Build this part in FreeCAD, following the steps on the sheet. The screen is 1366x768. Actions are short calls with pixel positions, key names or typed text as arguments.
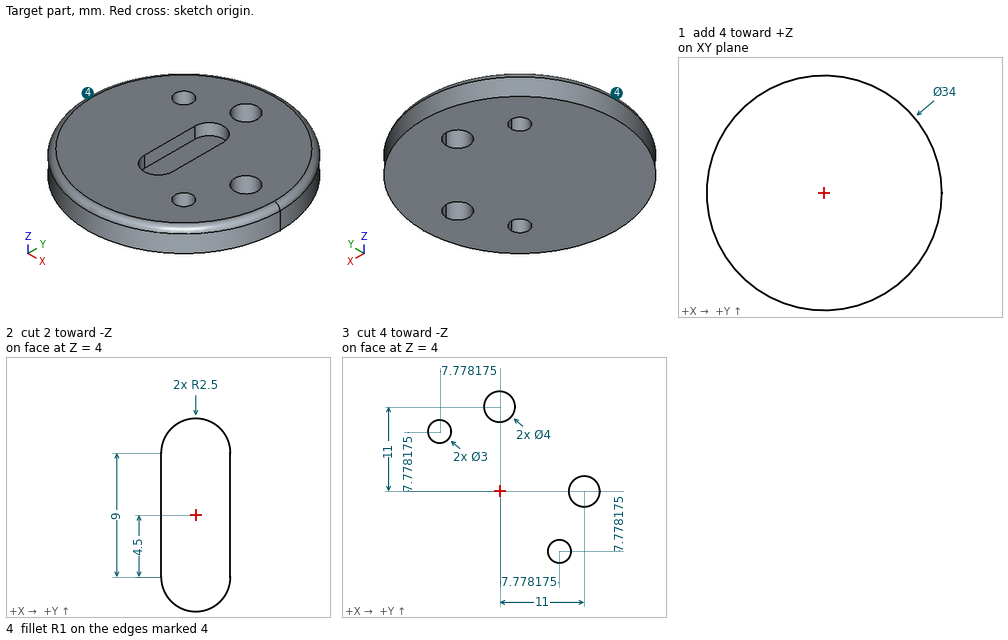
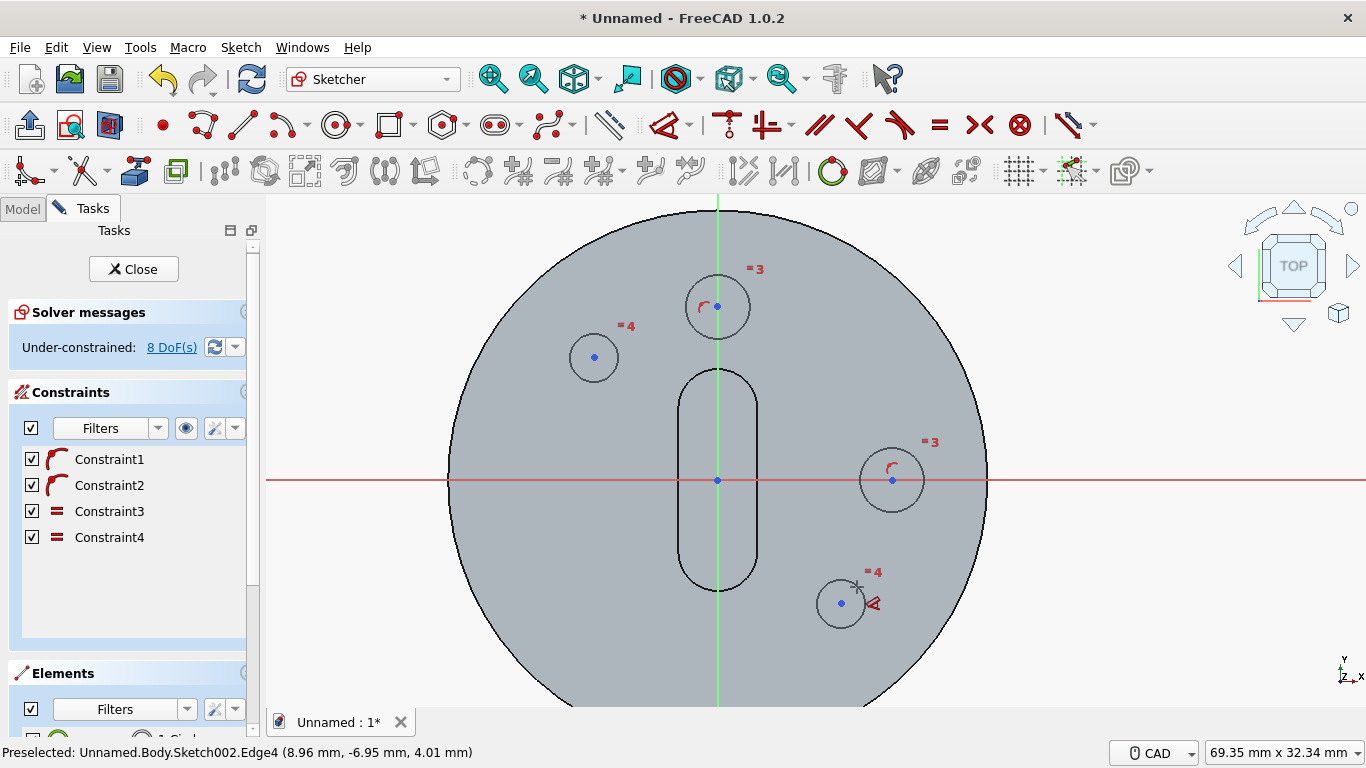
click(740, 284)
click(762, 261)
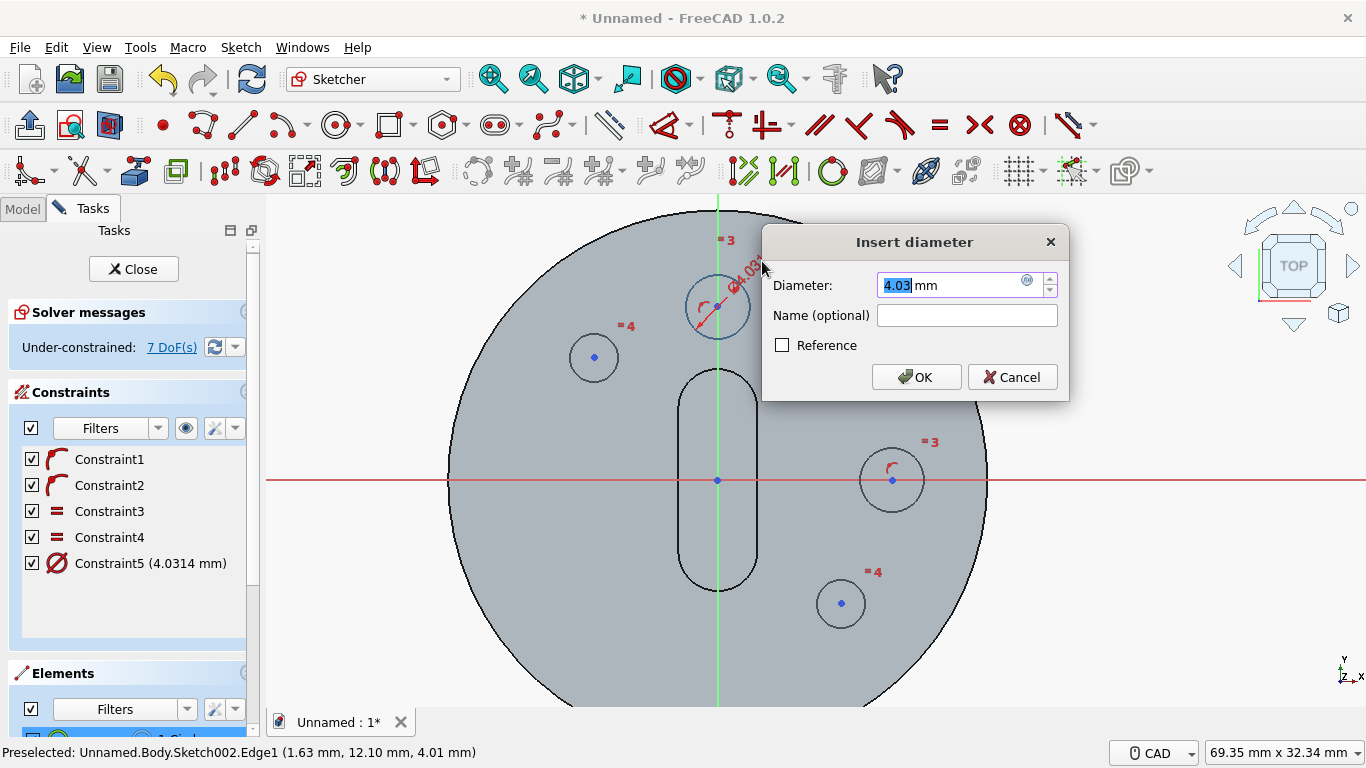
text(4)
key(Return)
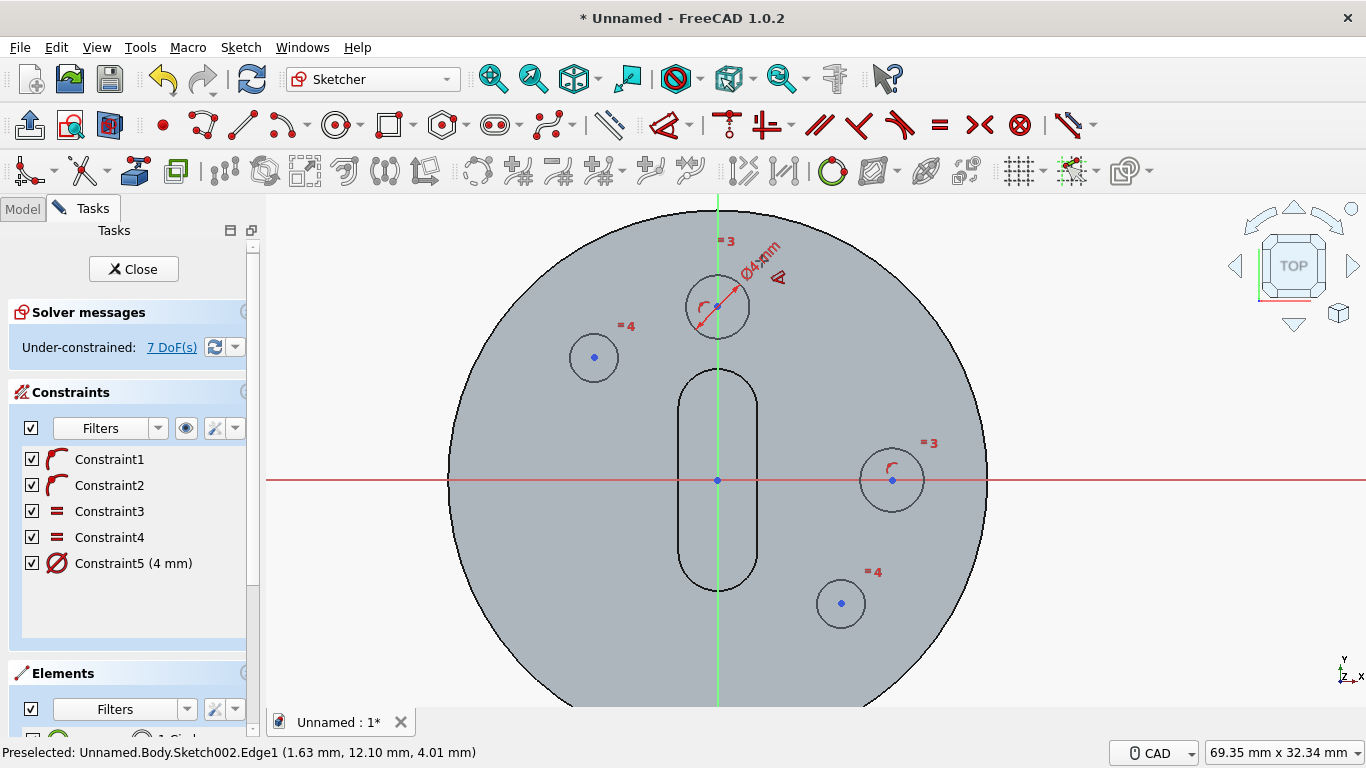
click(611, 341)
click(634, 318)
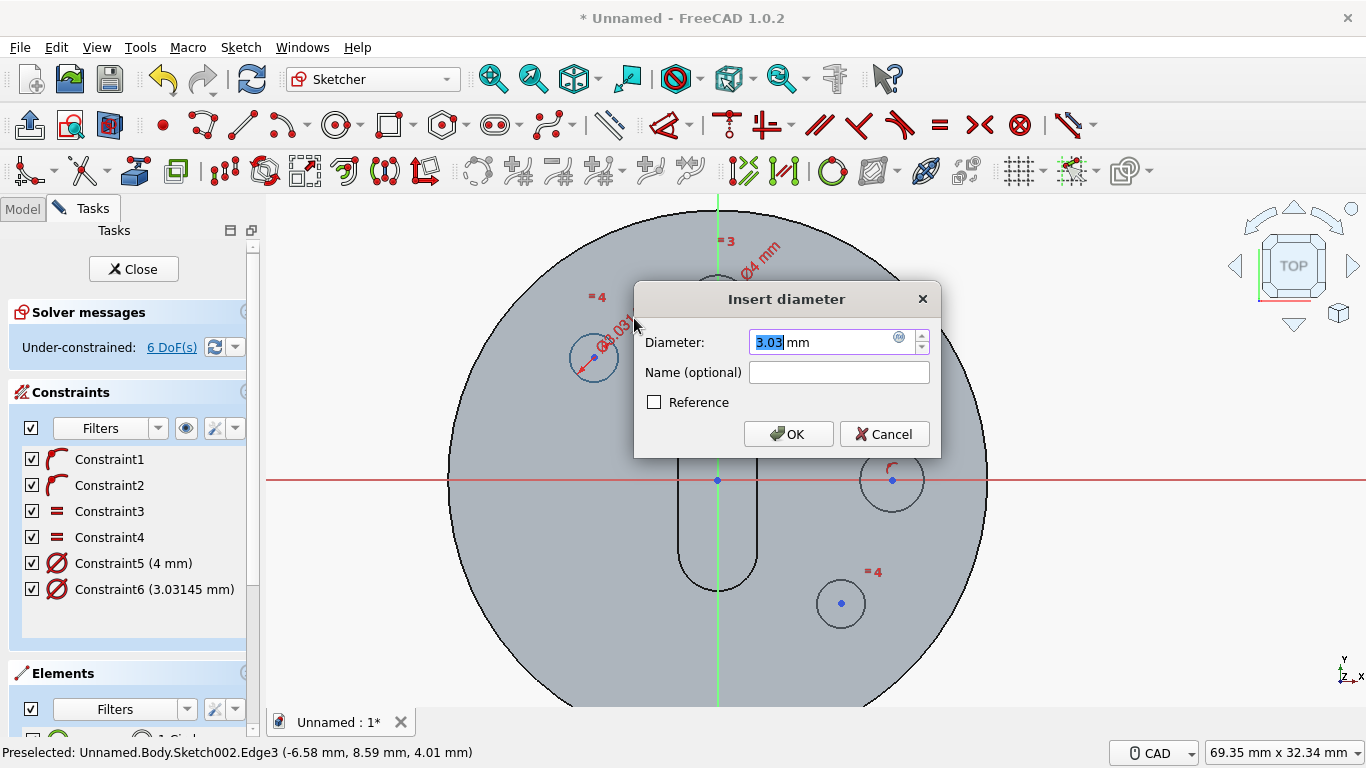
text(3)
key(Return)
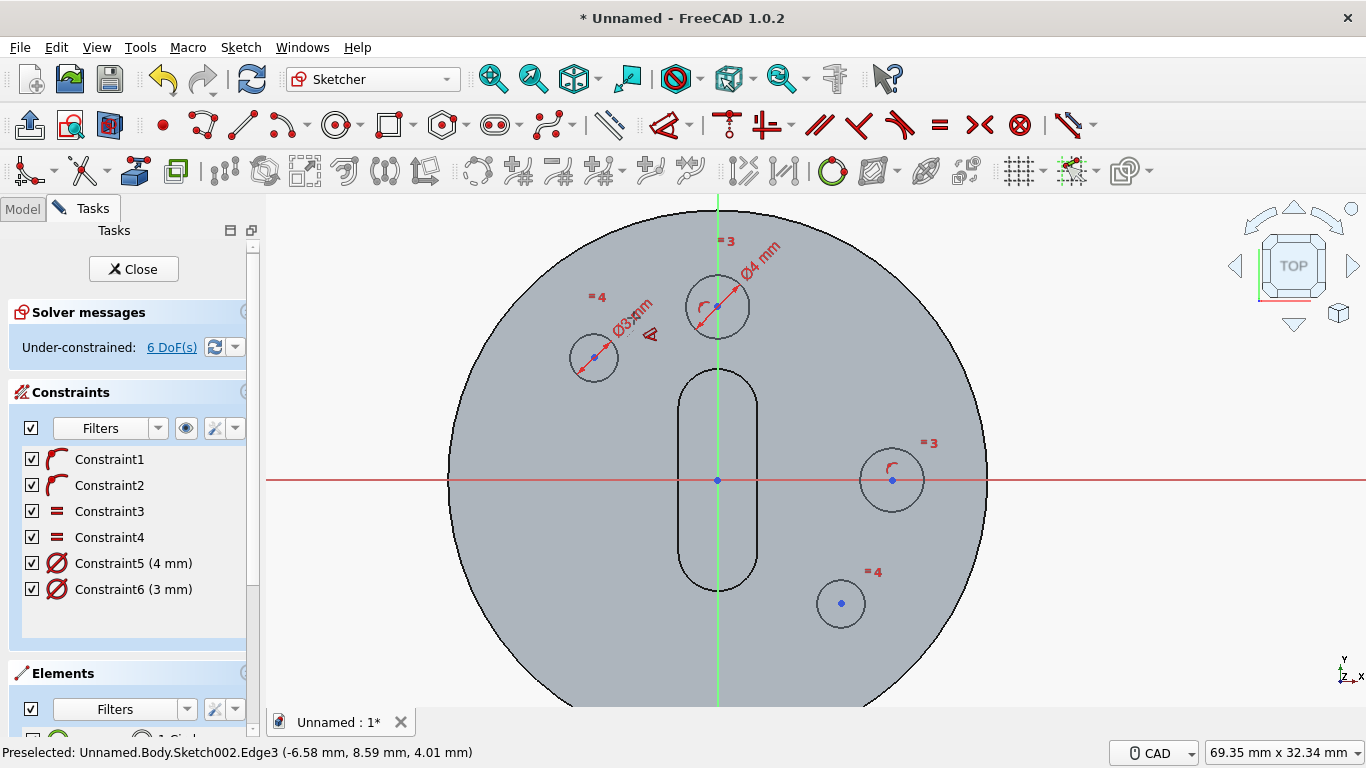
click(718, 307)
click(684, 394)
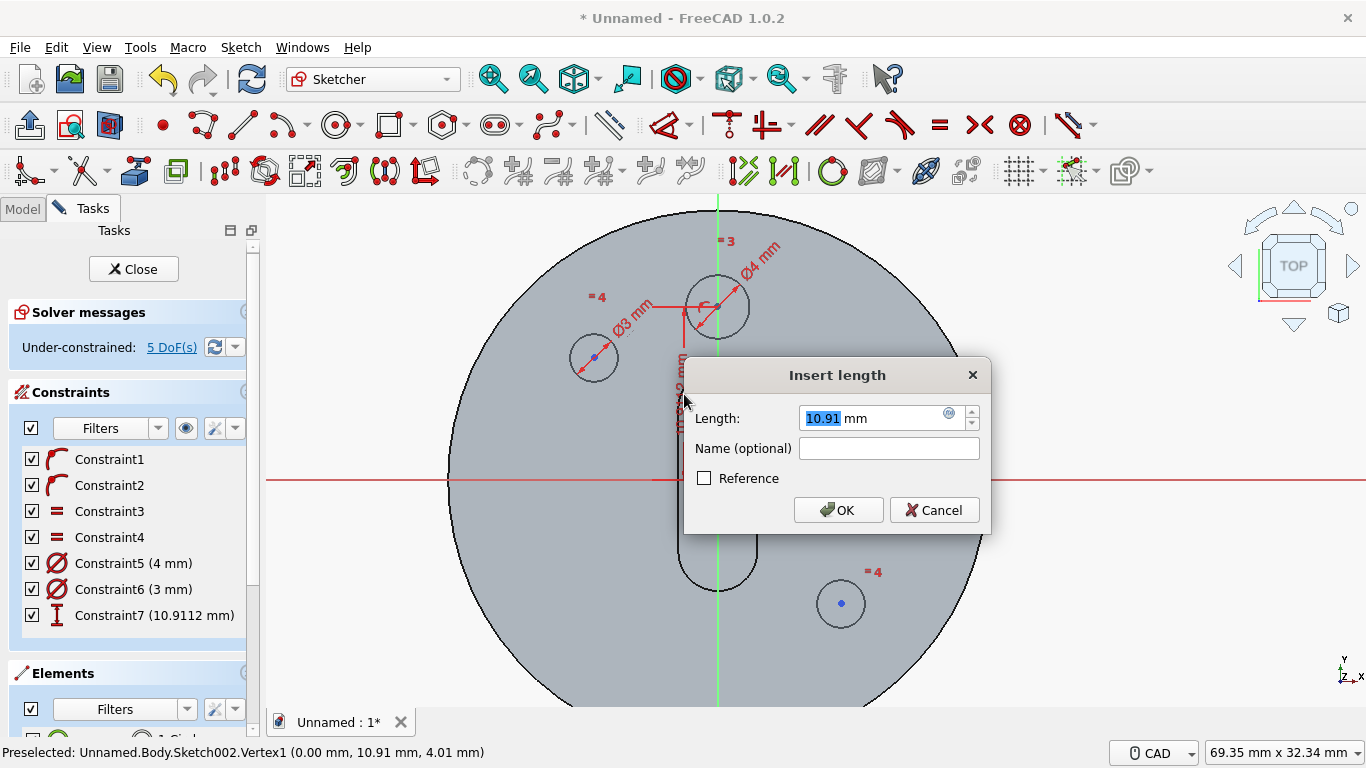
text(11)
key(Return)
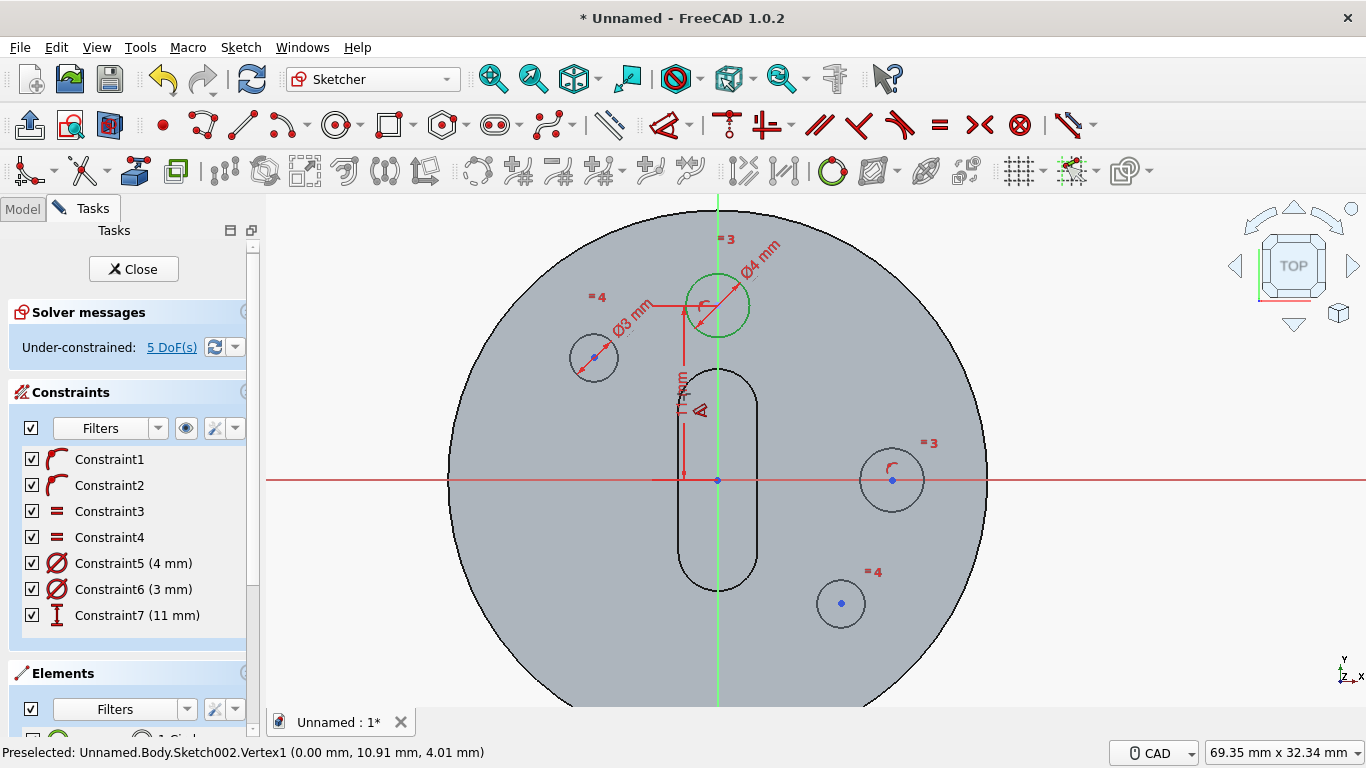
click(892, 480)
click(805, 514)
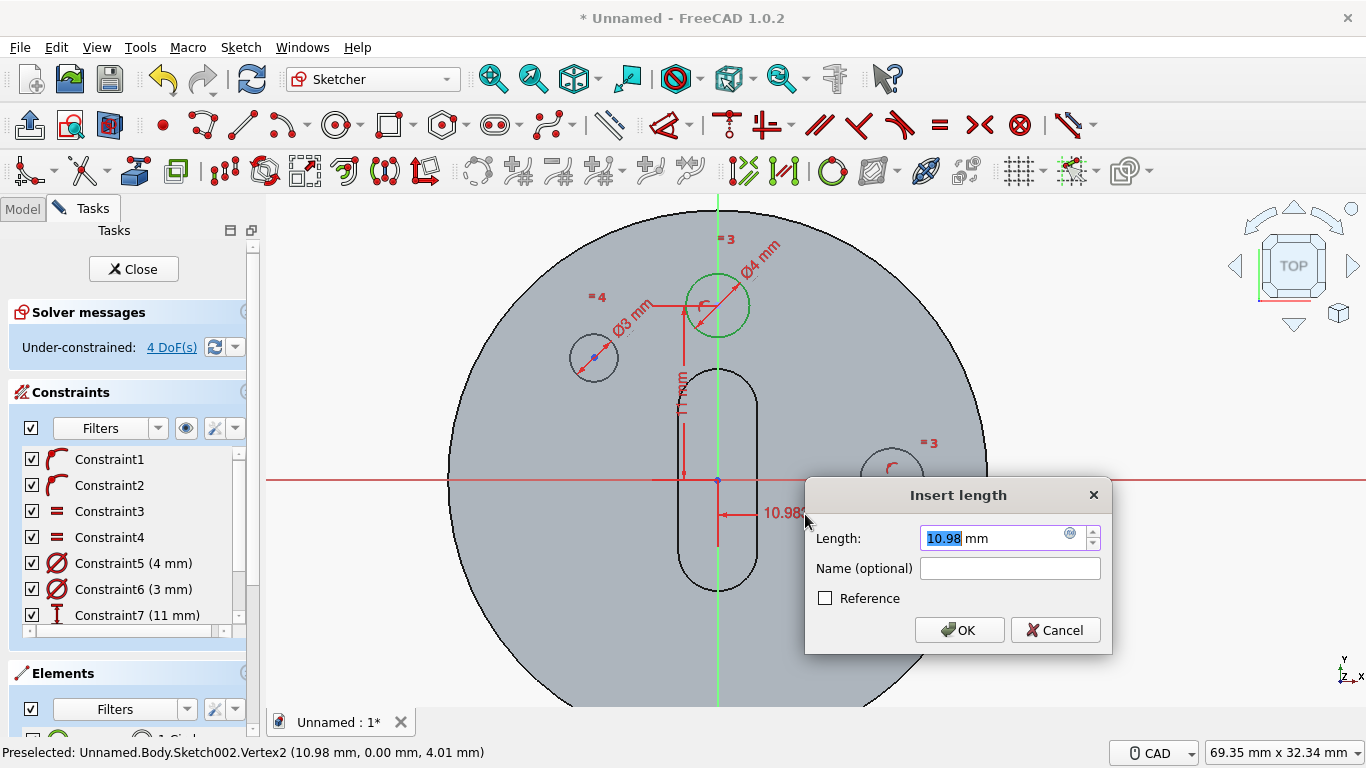
text(11)
key(Return)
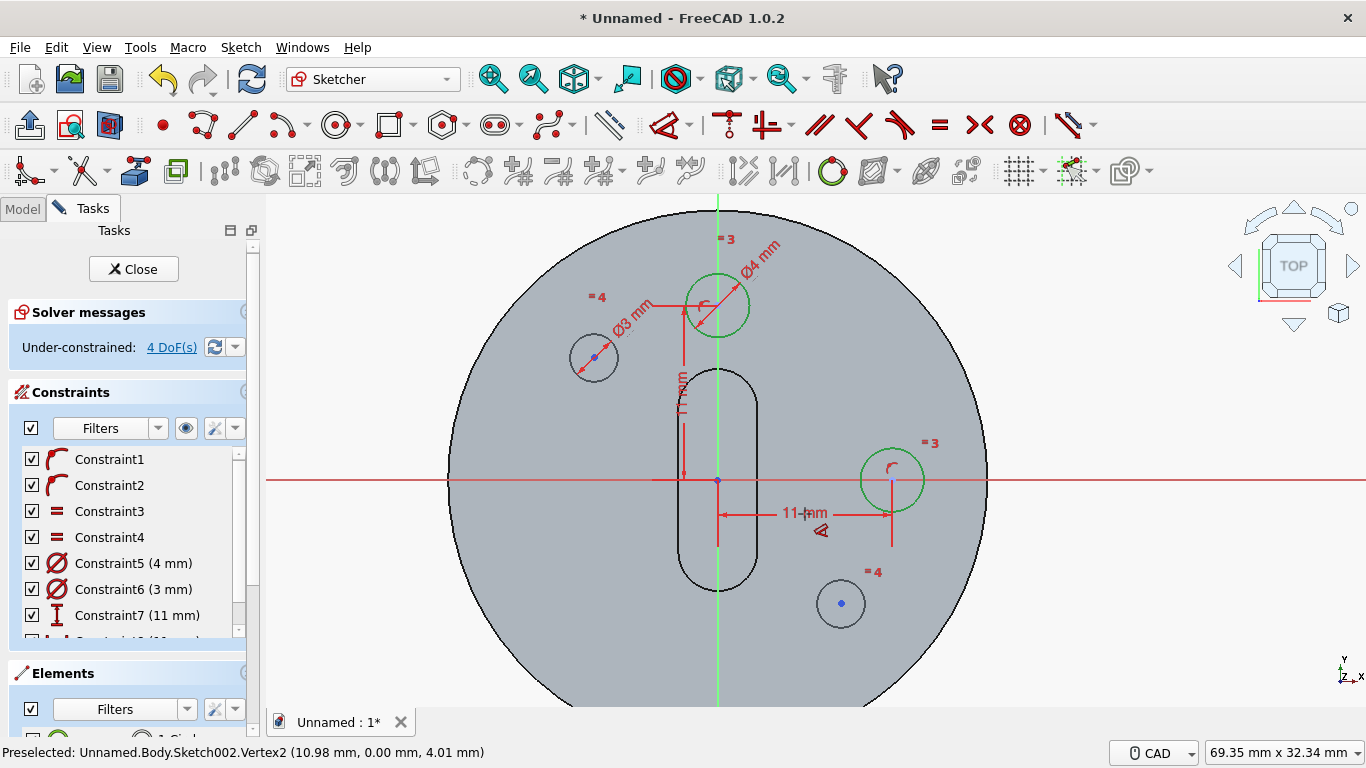
click(594, 358)
click(656, 514)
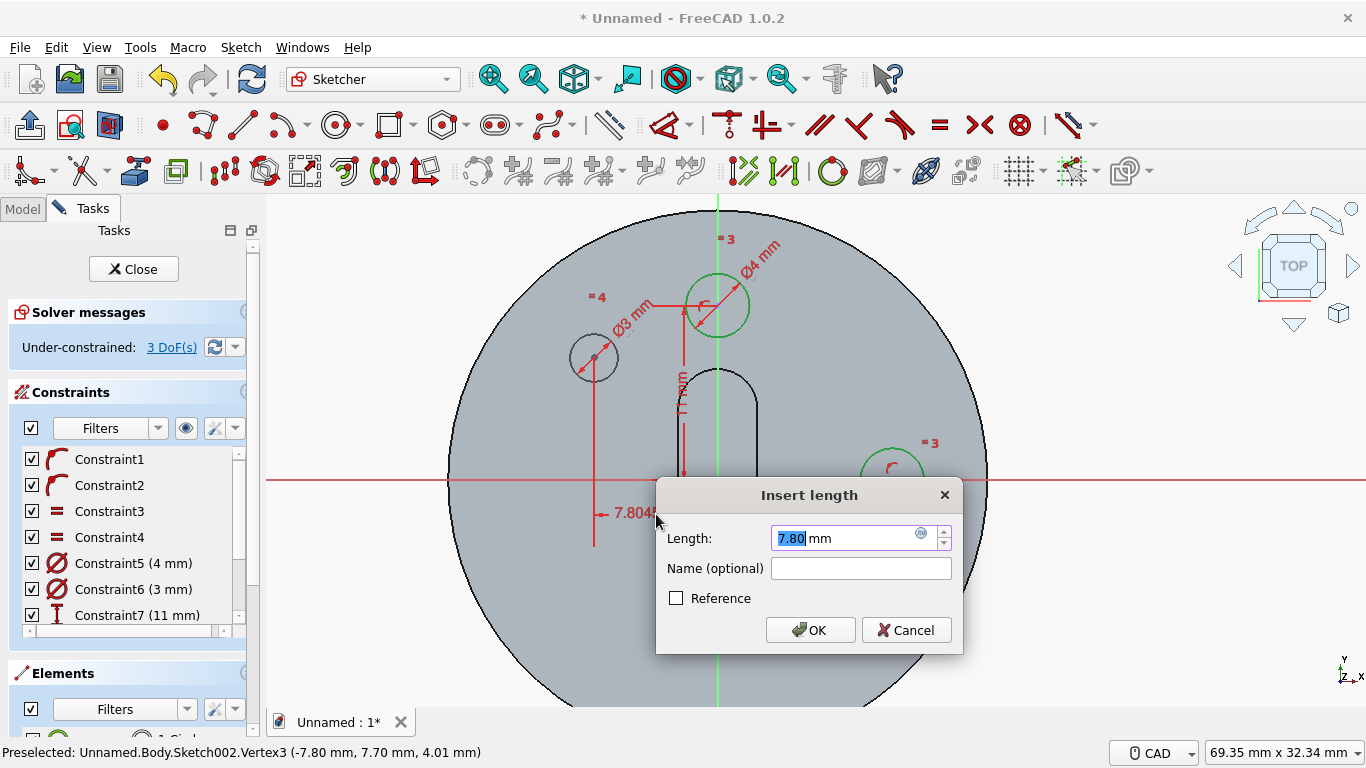
text(7.778175)
key(Return)